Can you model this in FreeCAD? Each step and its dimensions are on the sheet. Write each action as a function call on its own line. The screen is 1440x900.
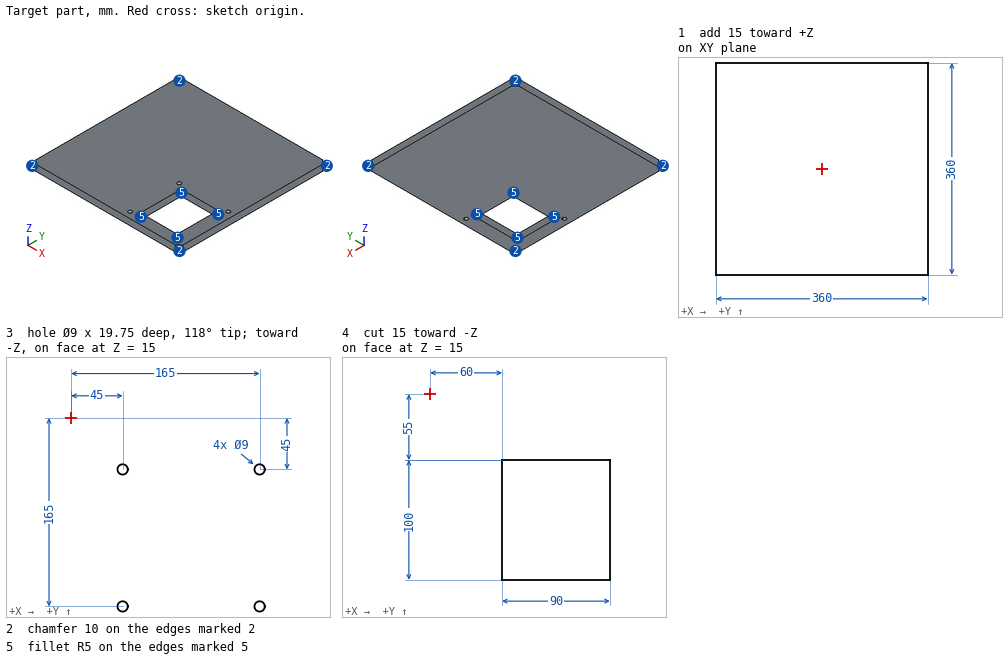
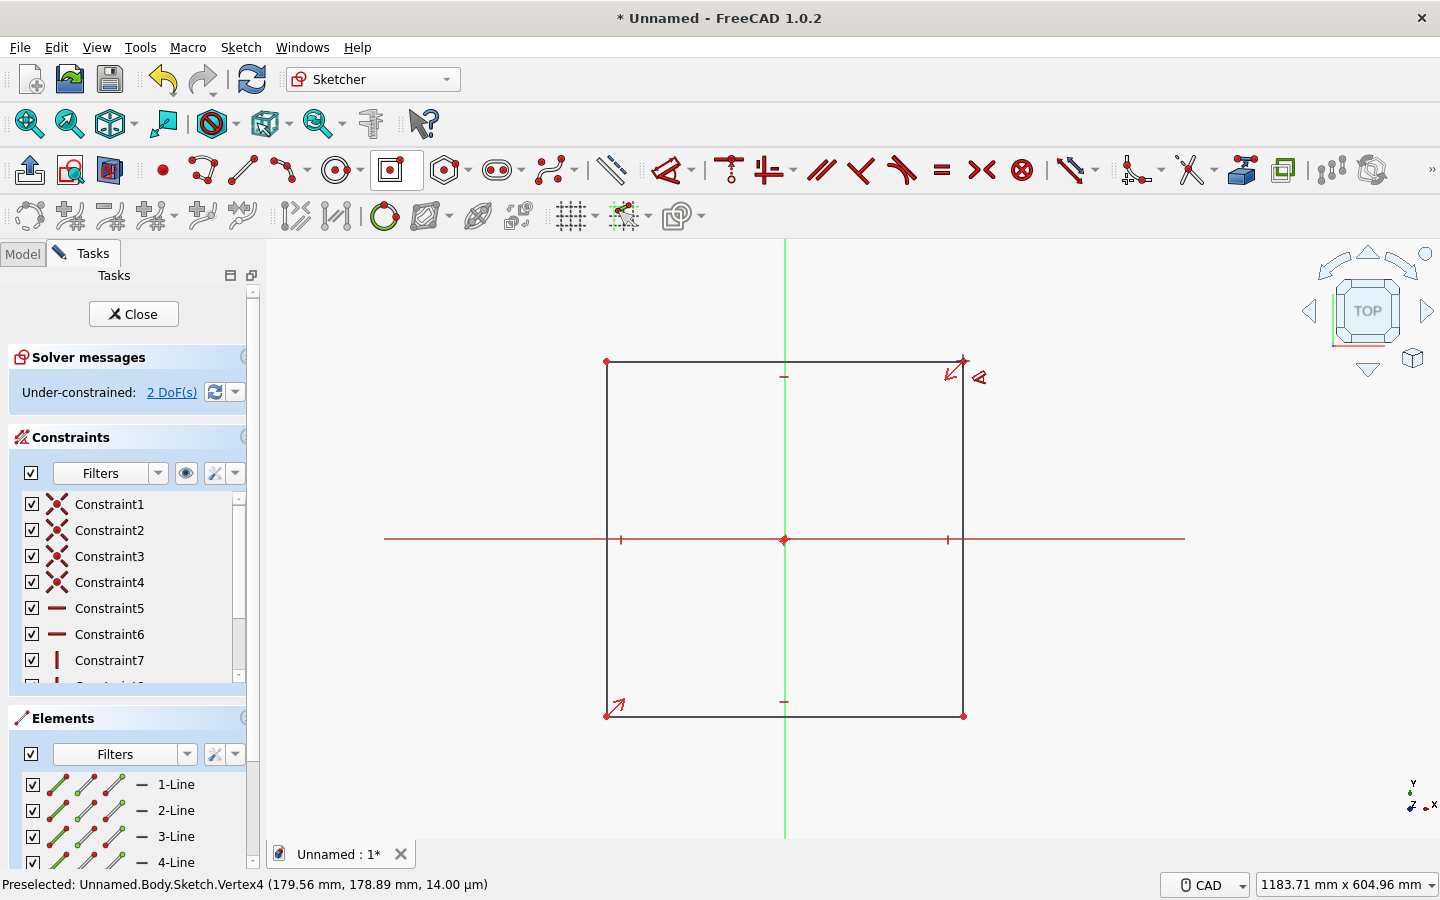
click(714, 717)
click(703, 751)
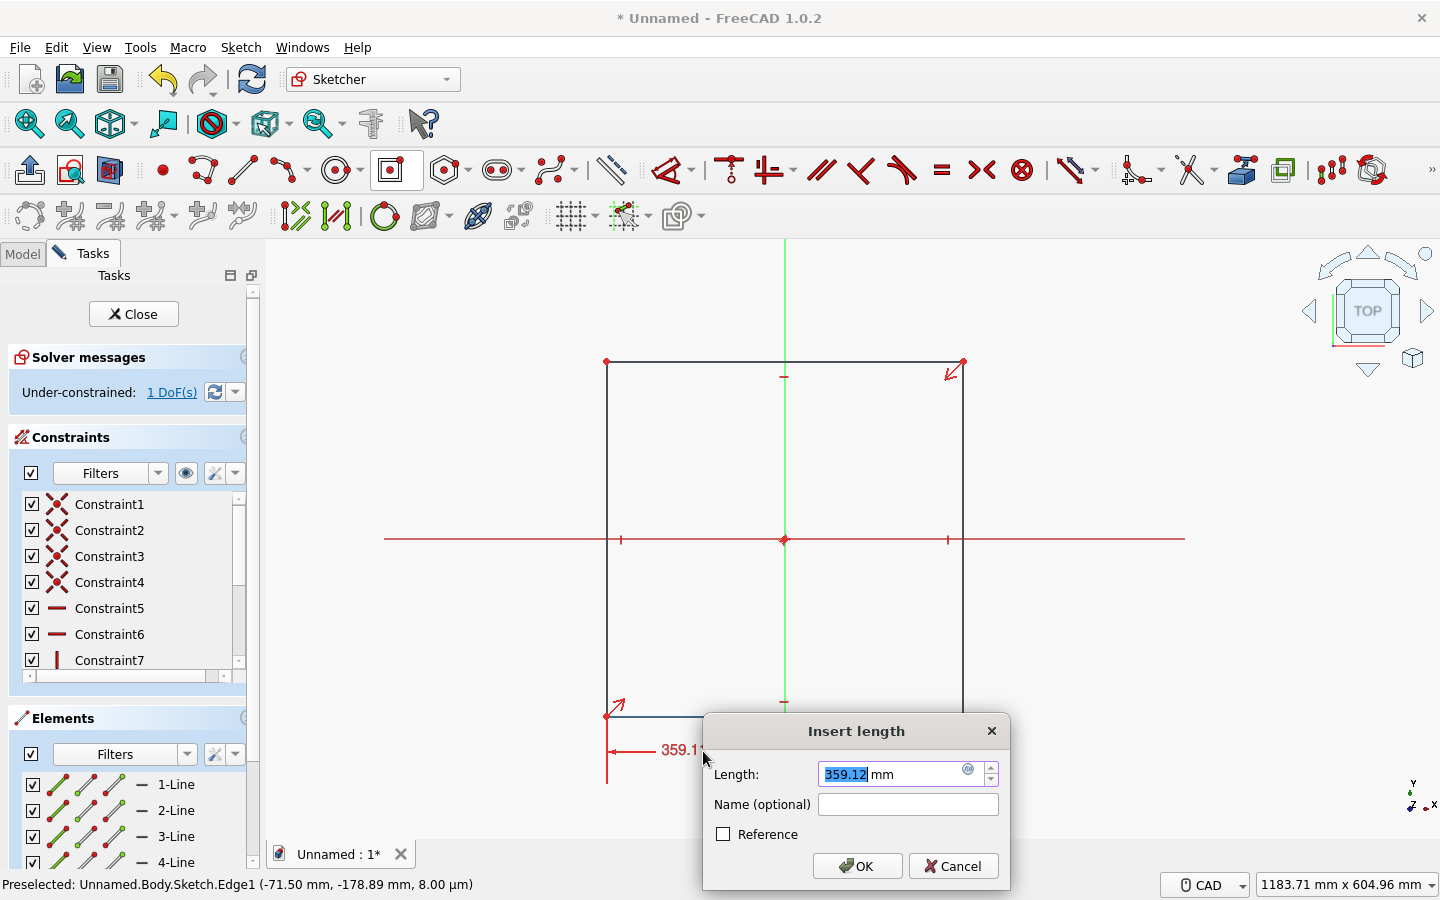
text(360)
key(Return)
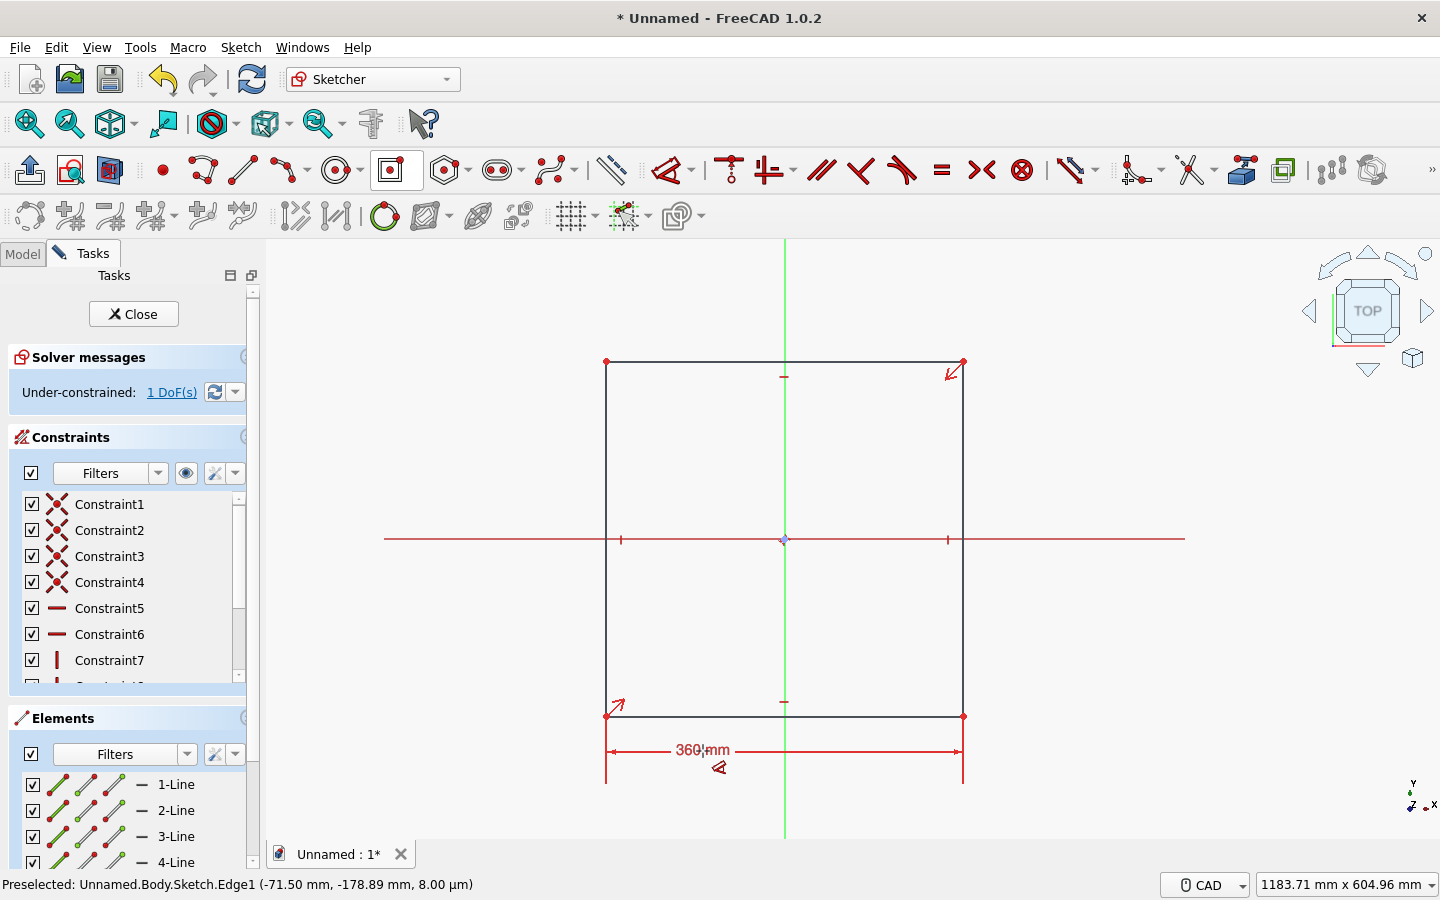
click(963, 610)
click(997, 458)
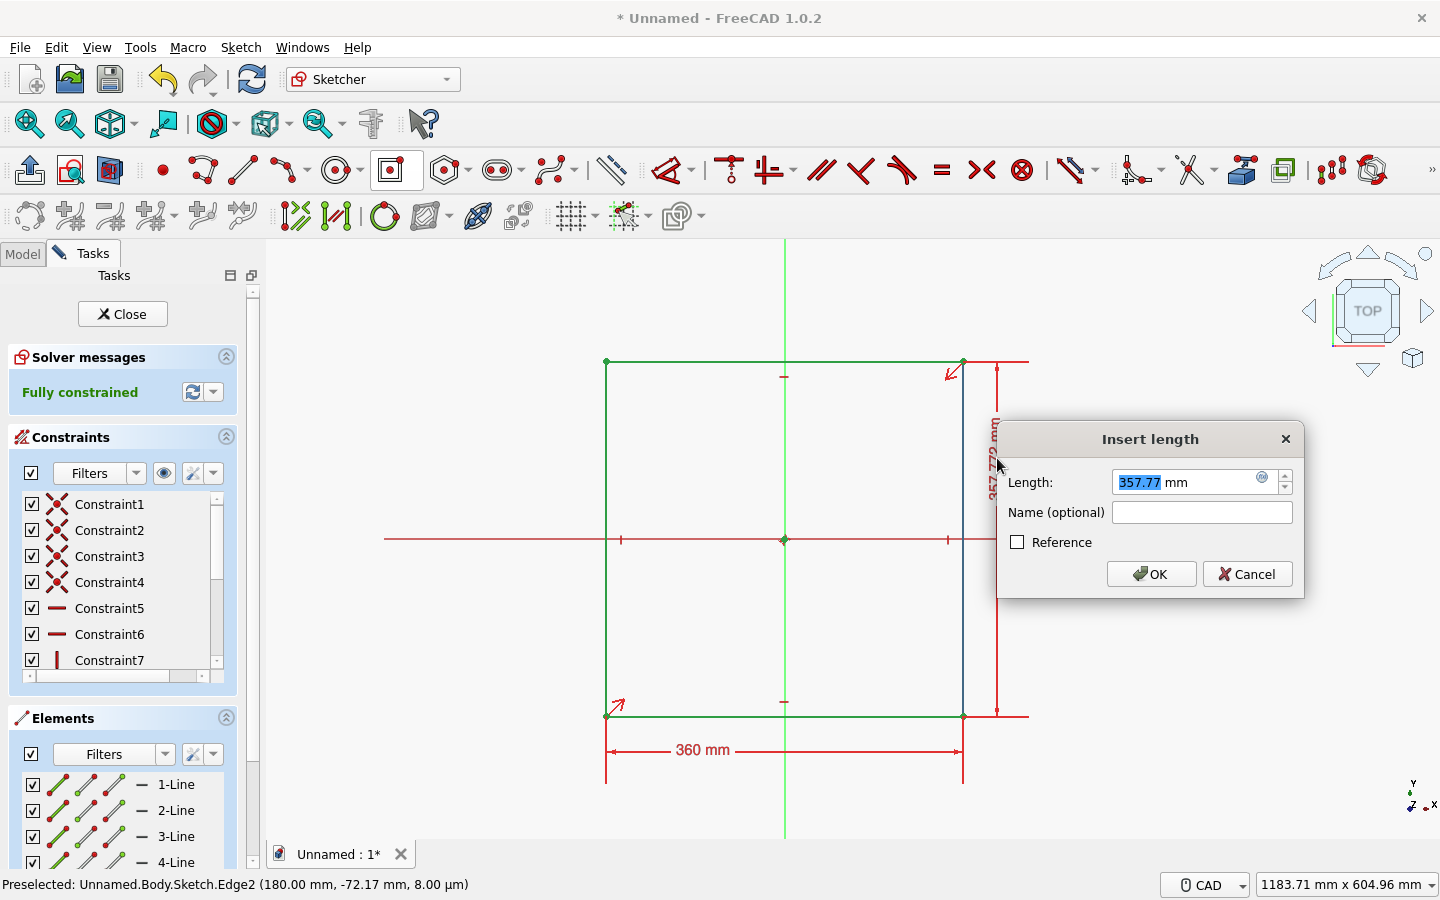
text(360)
key(Return)
key(Escape)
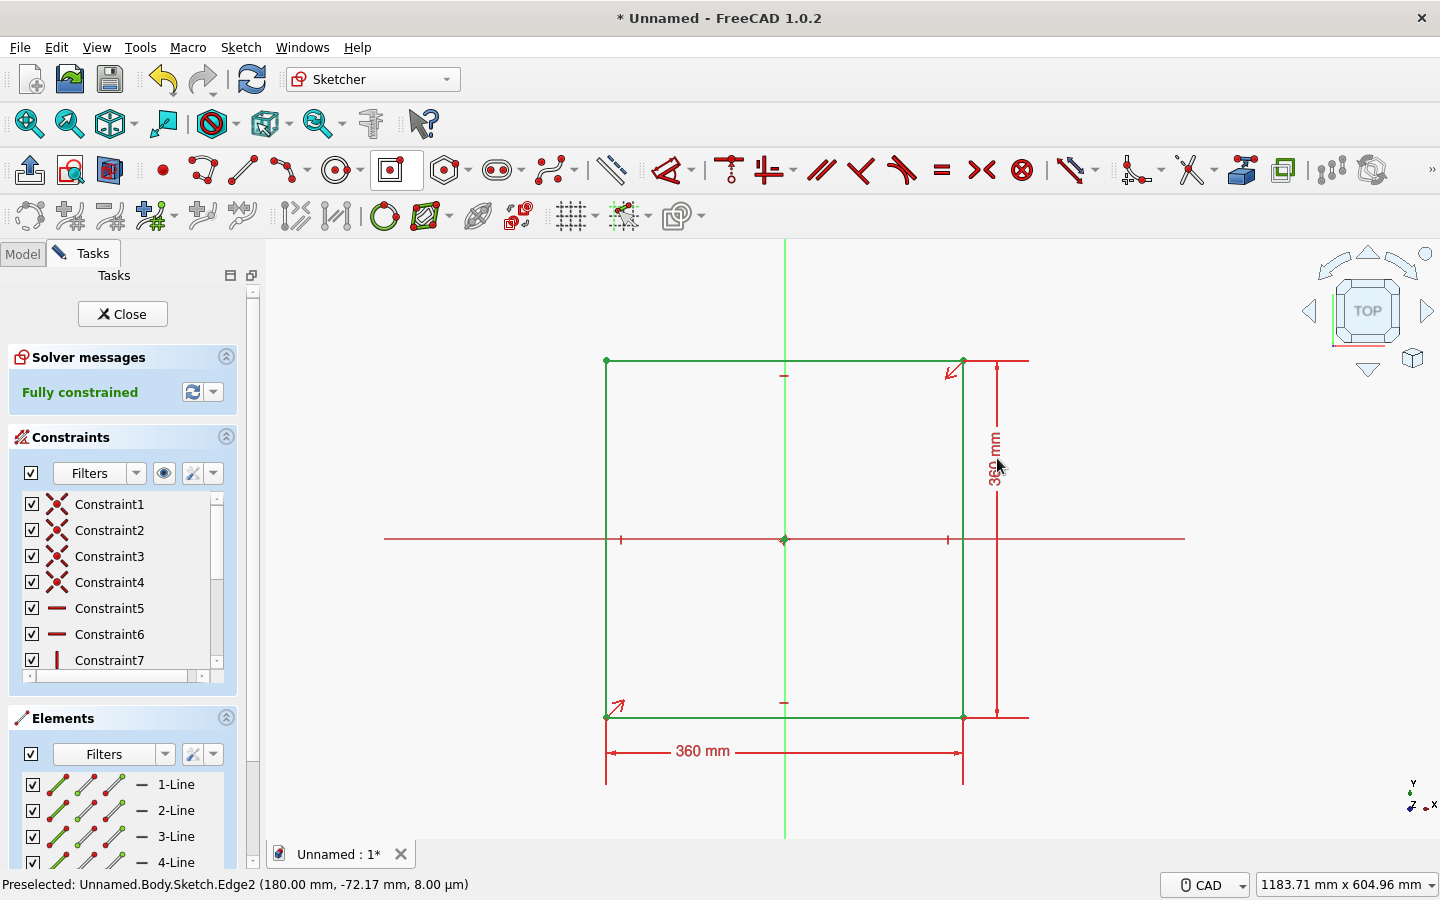
click(123, 314)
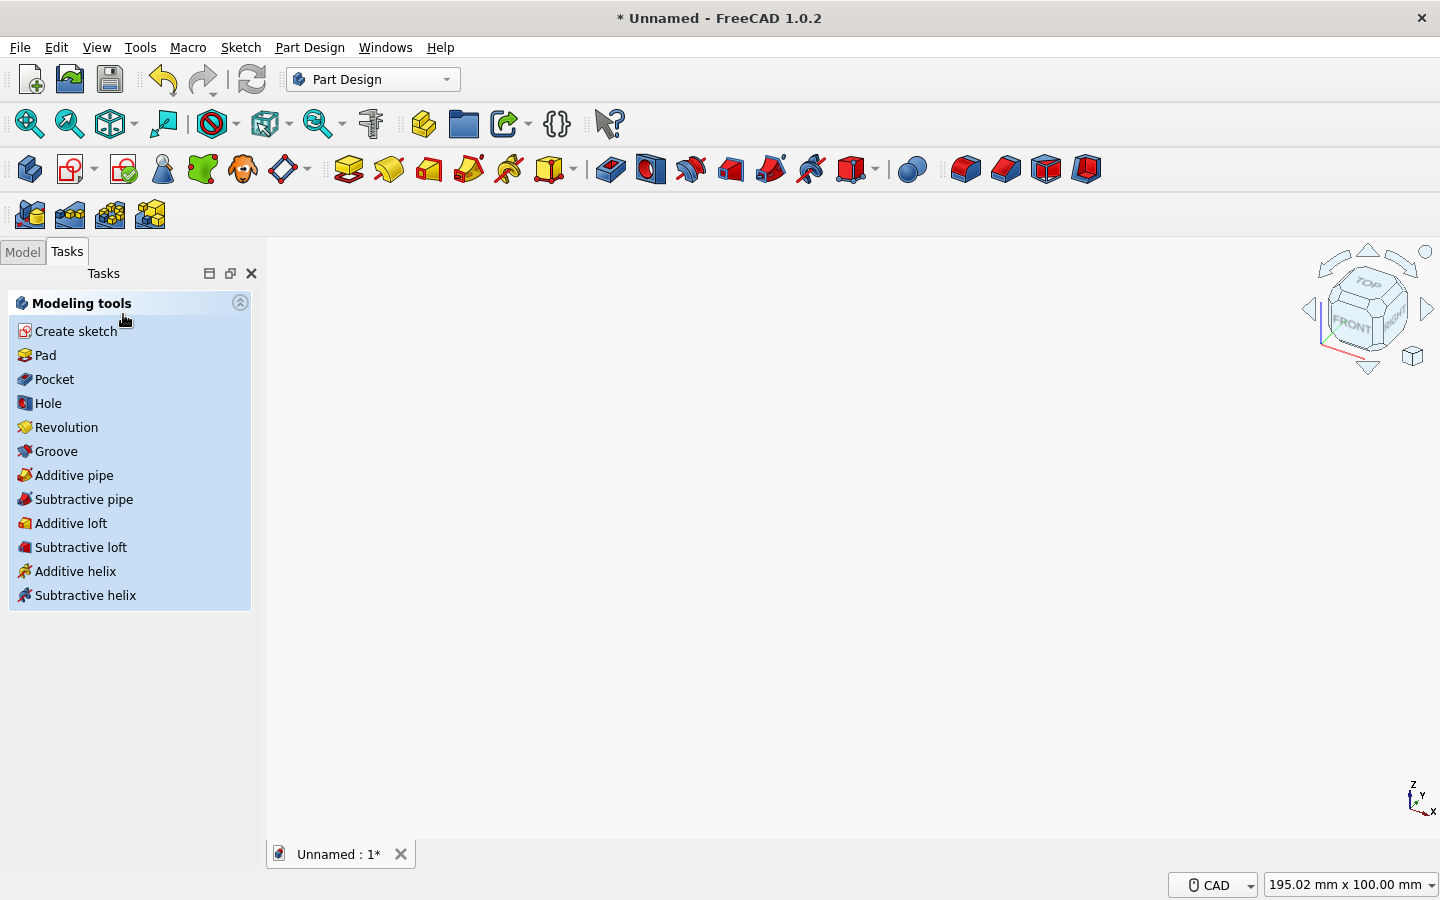
click(350, 170)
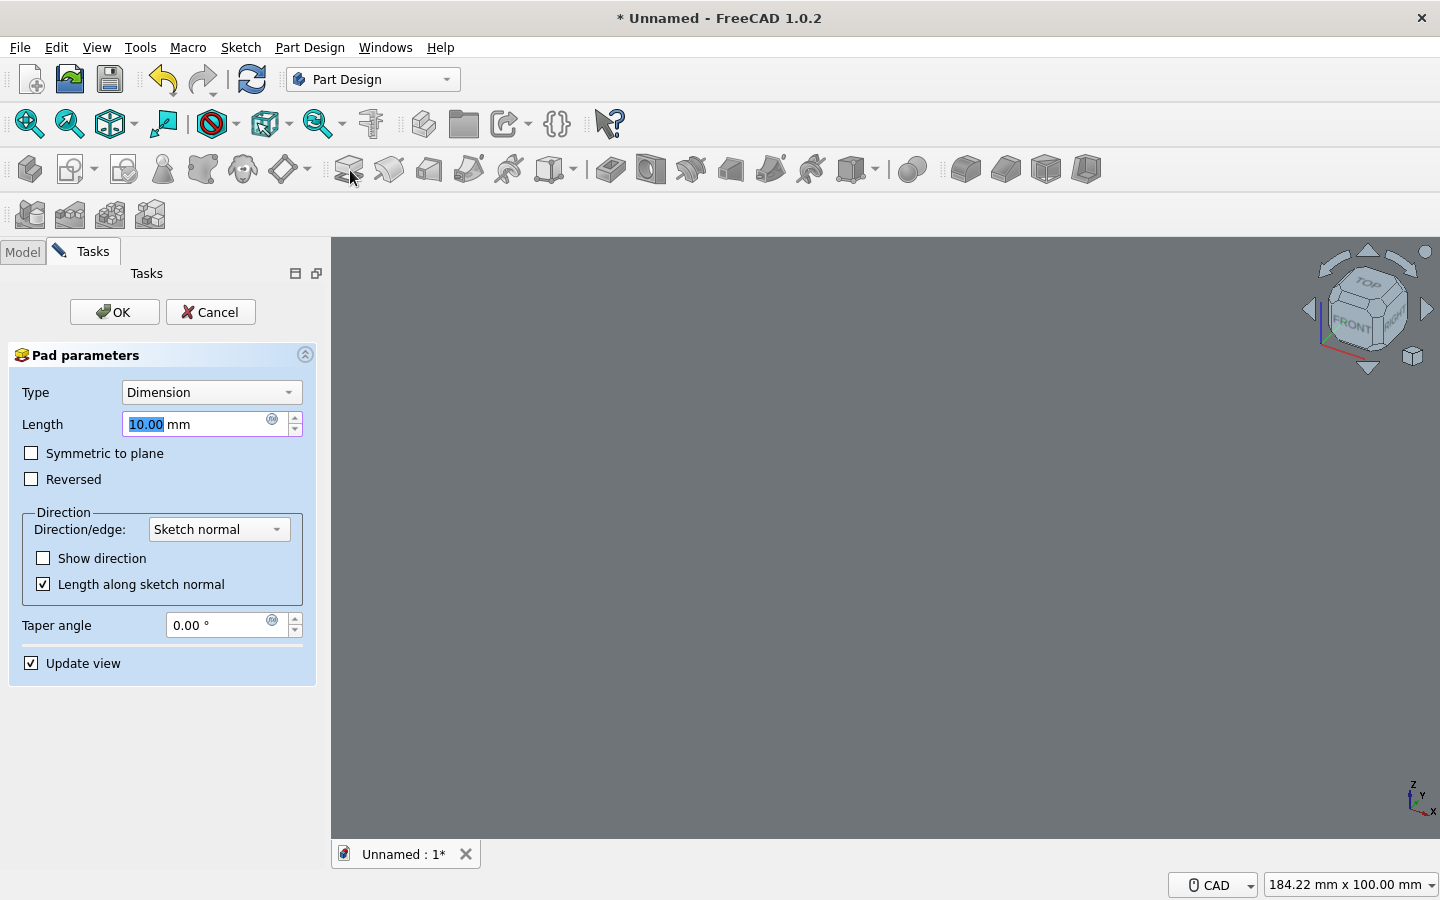
text(15)
key(Tab)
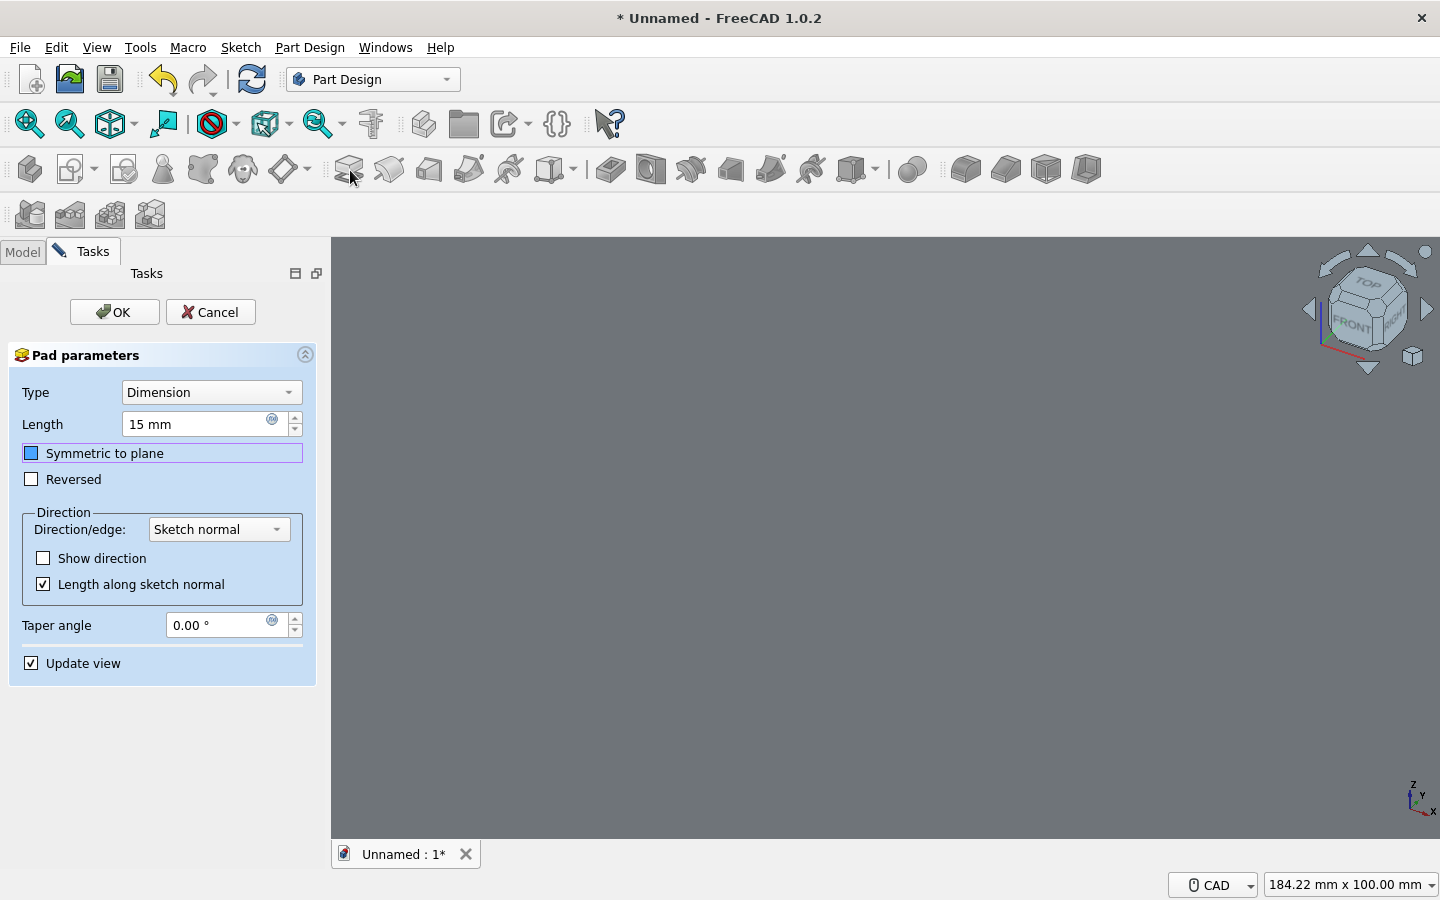
click(115, 312)